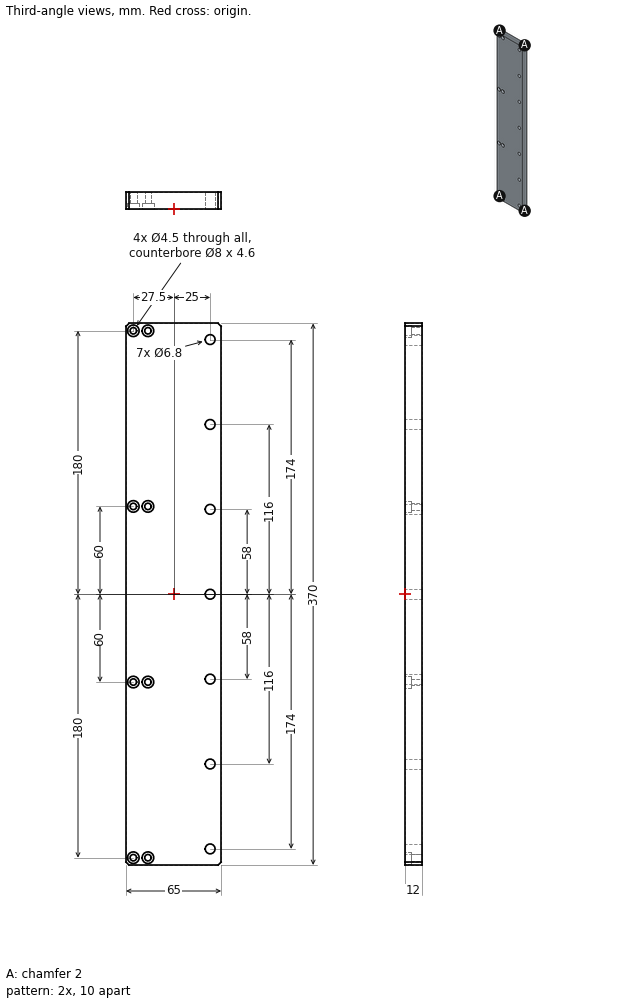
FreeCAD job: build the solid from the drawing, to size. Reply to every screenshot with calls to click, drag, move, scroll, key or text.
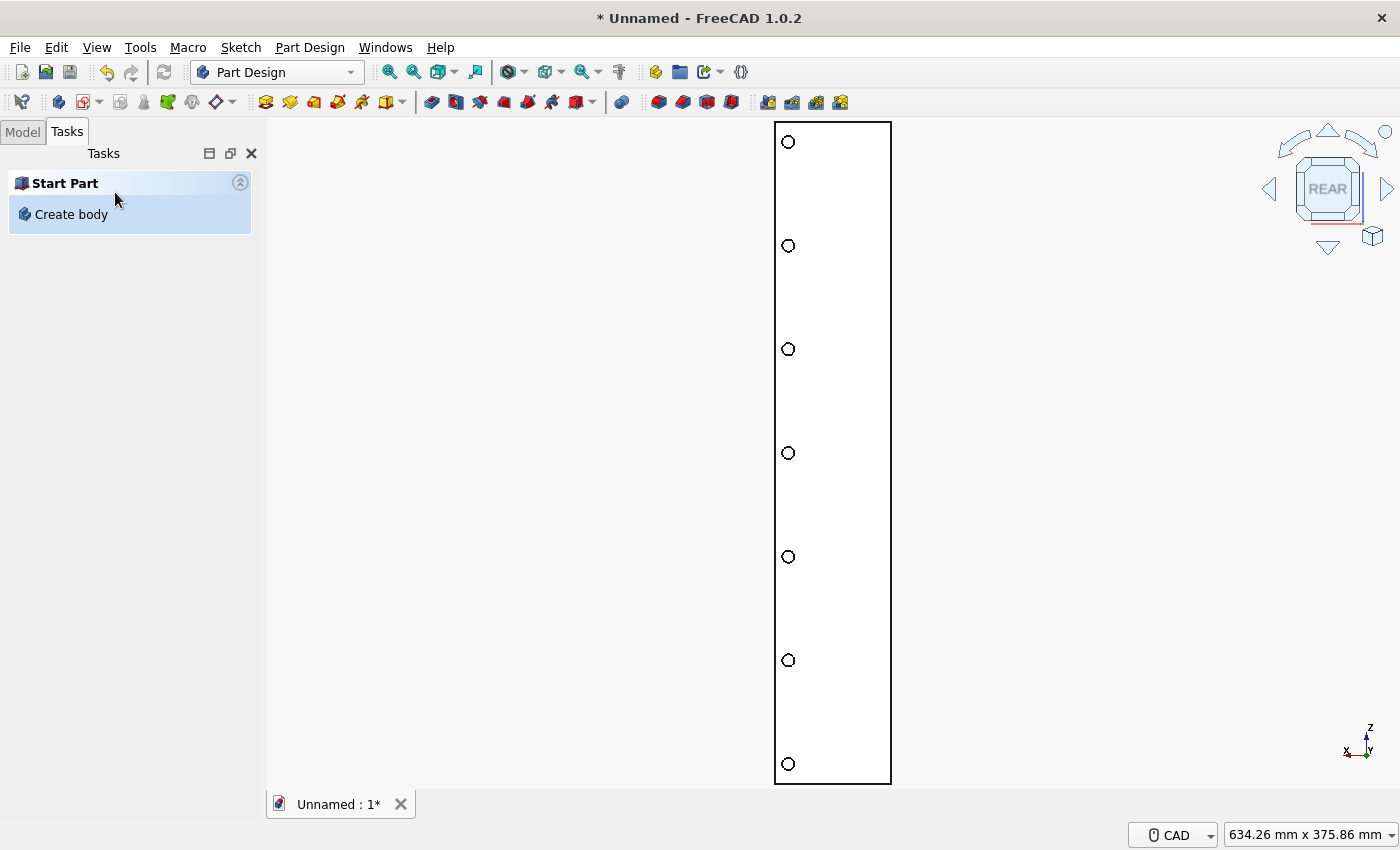
key(0)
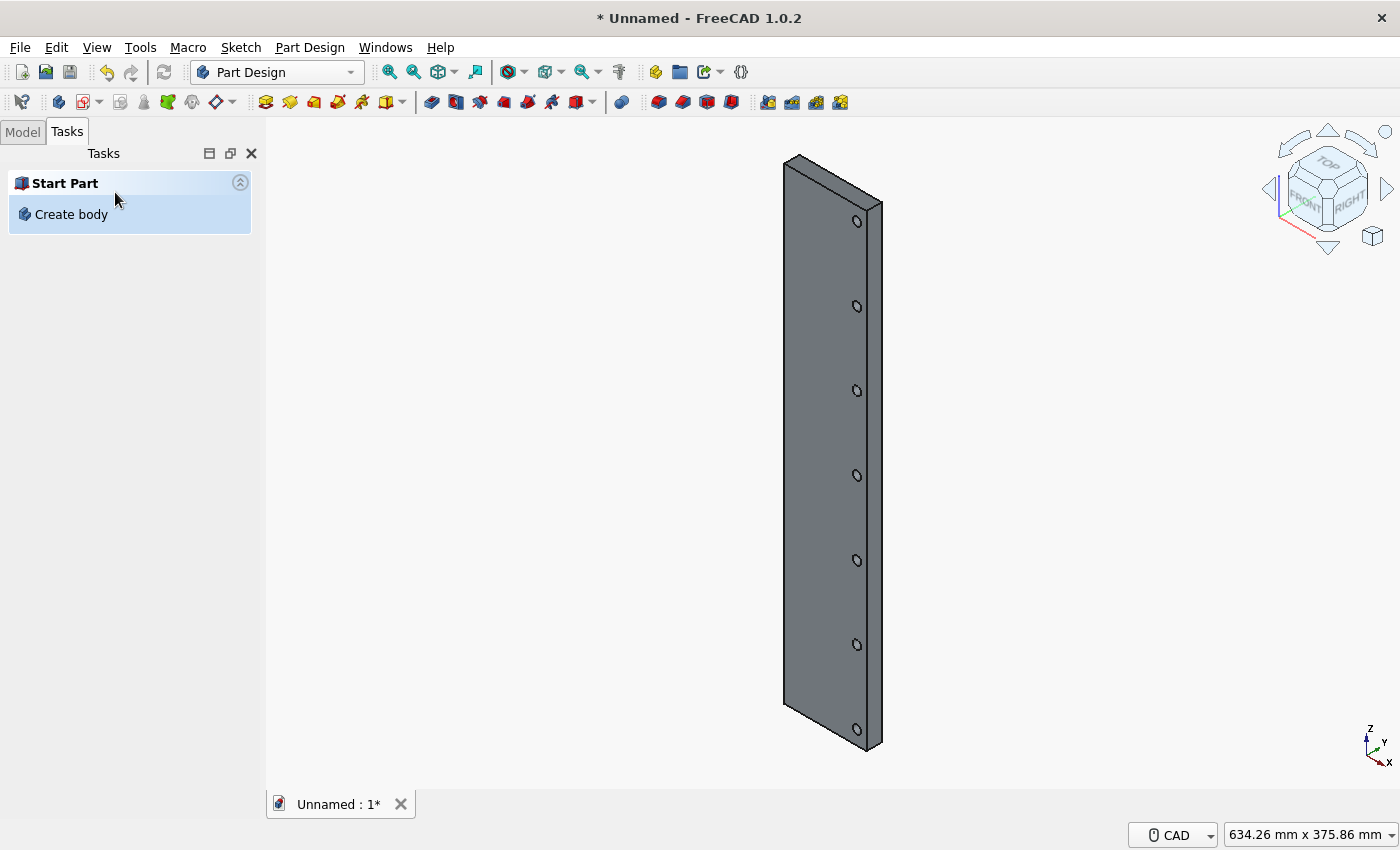
click(825, 225)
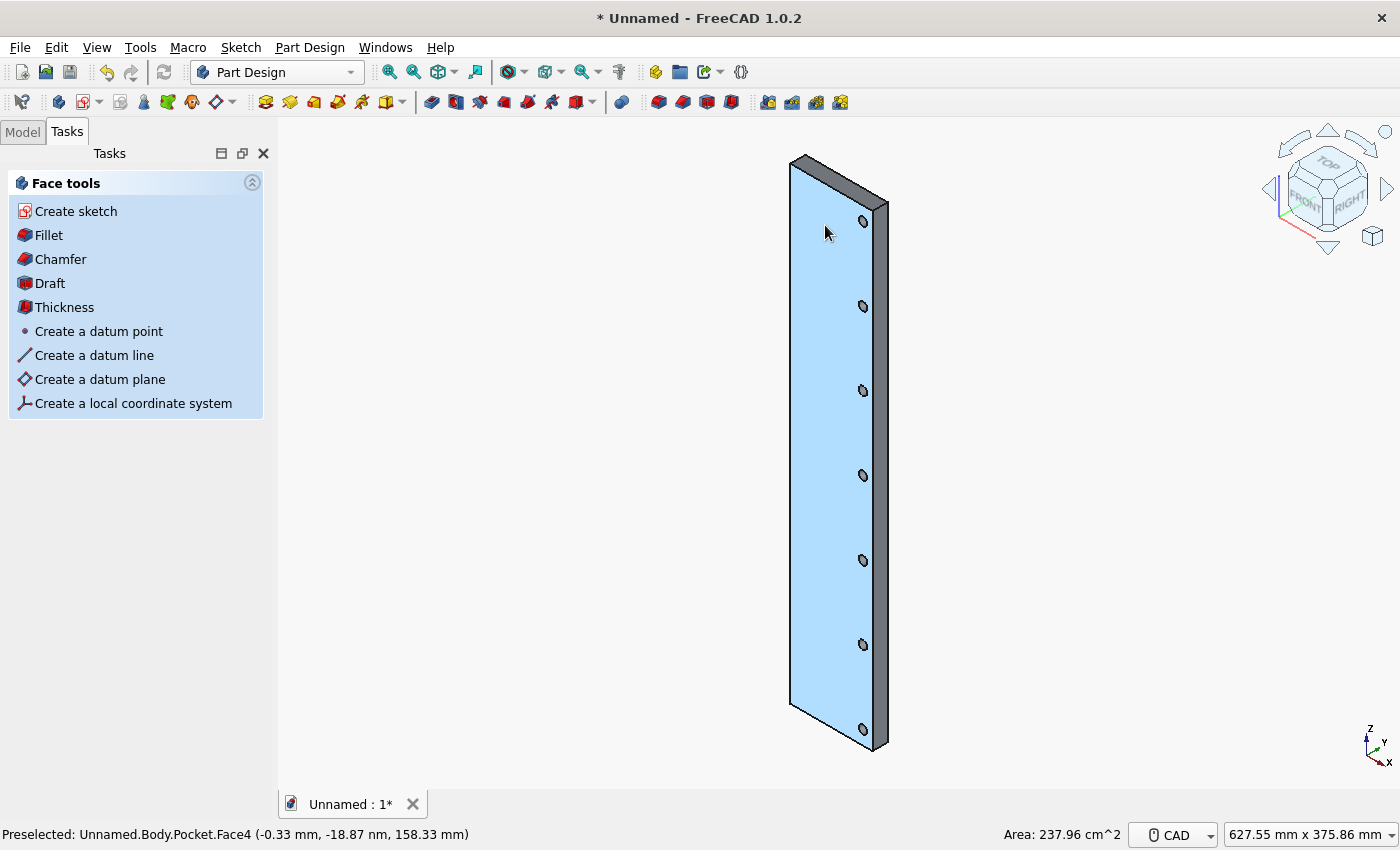
click(84, 102)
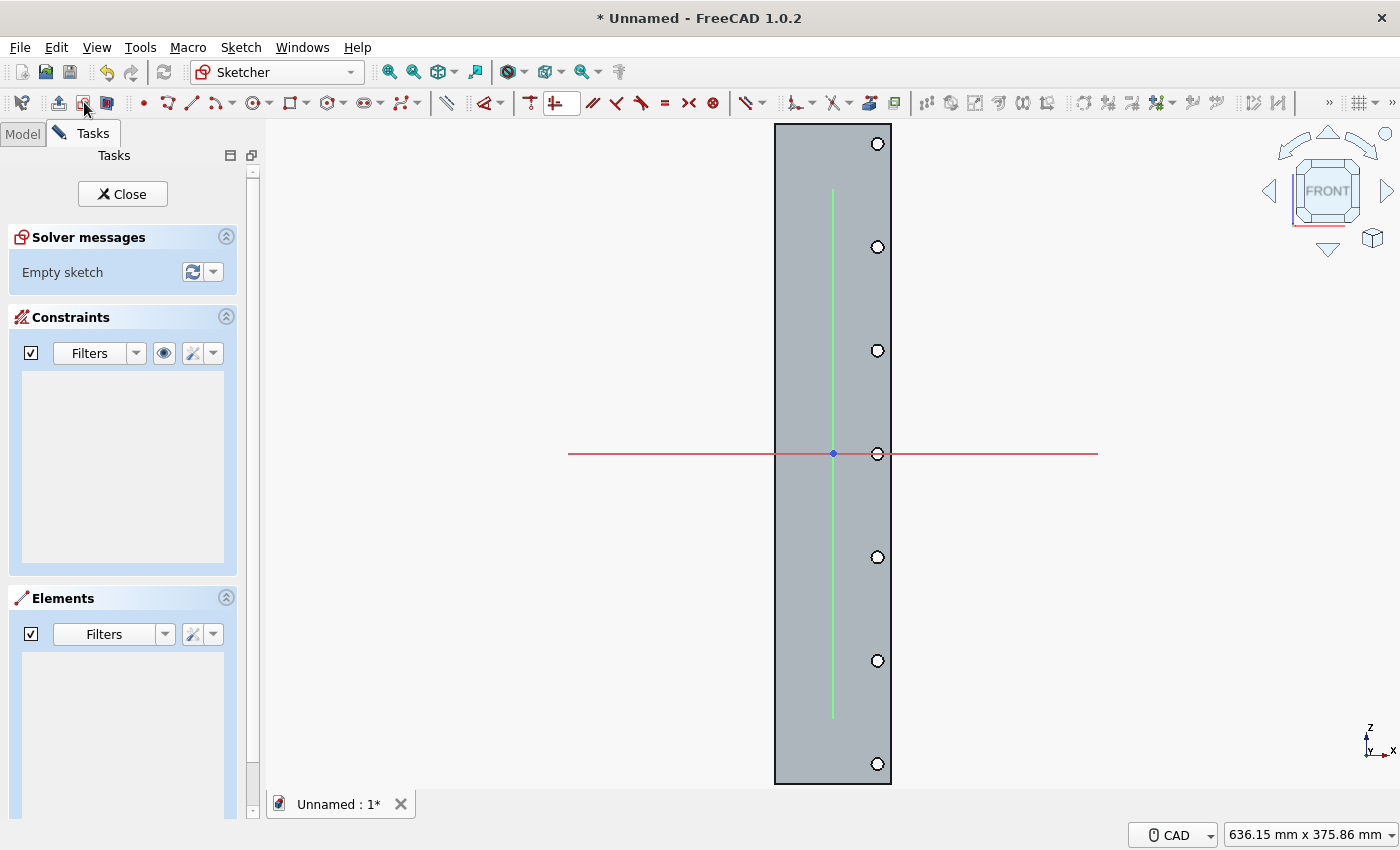
scroll(679, 454, down, 2)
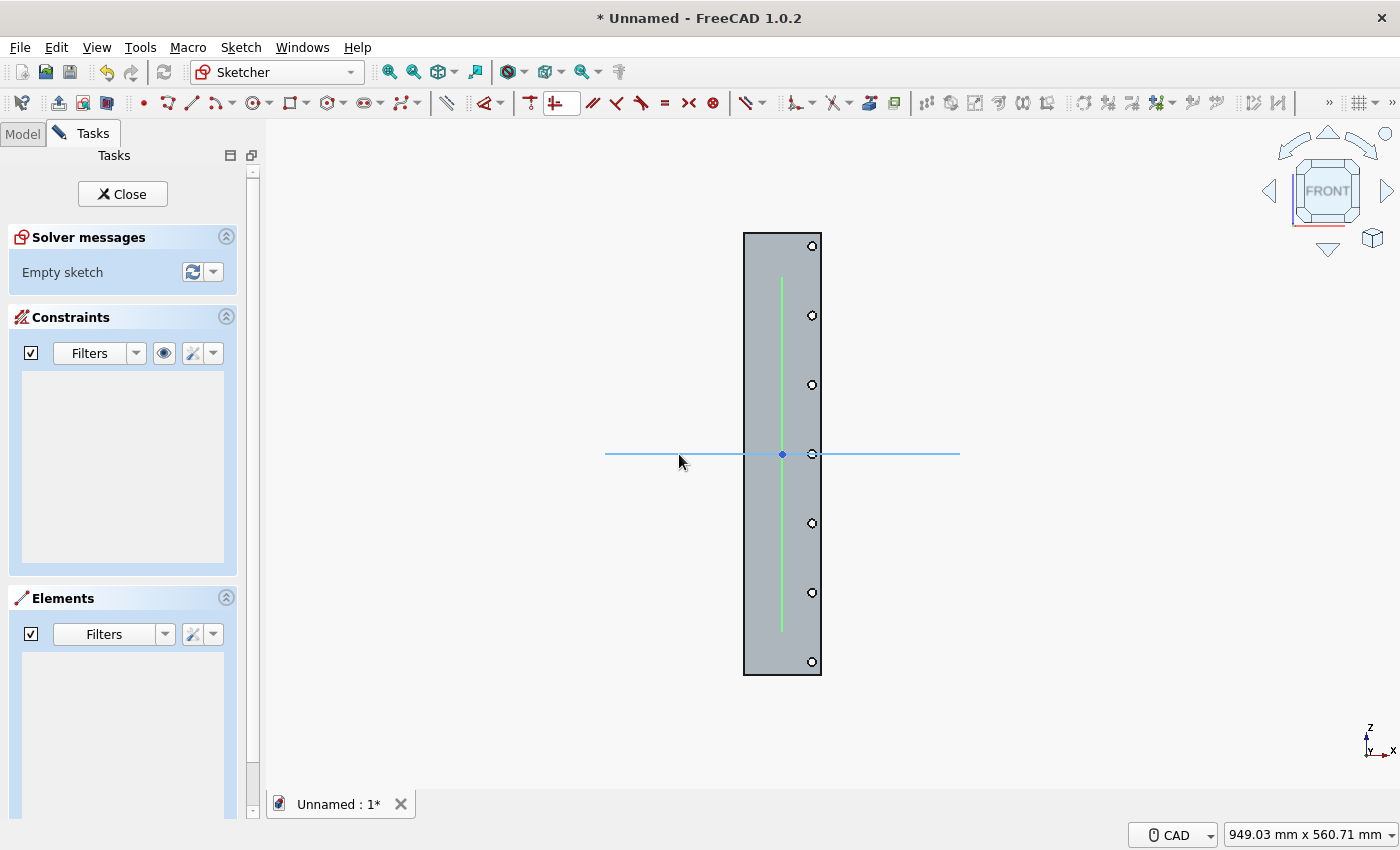
key(g)
key(c)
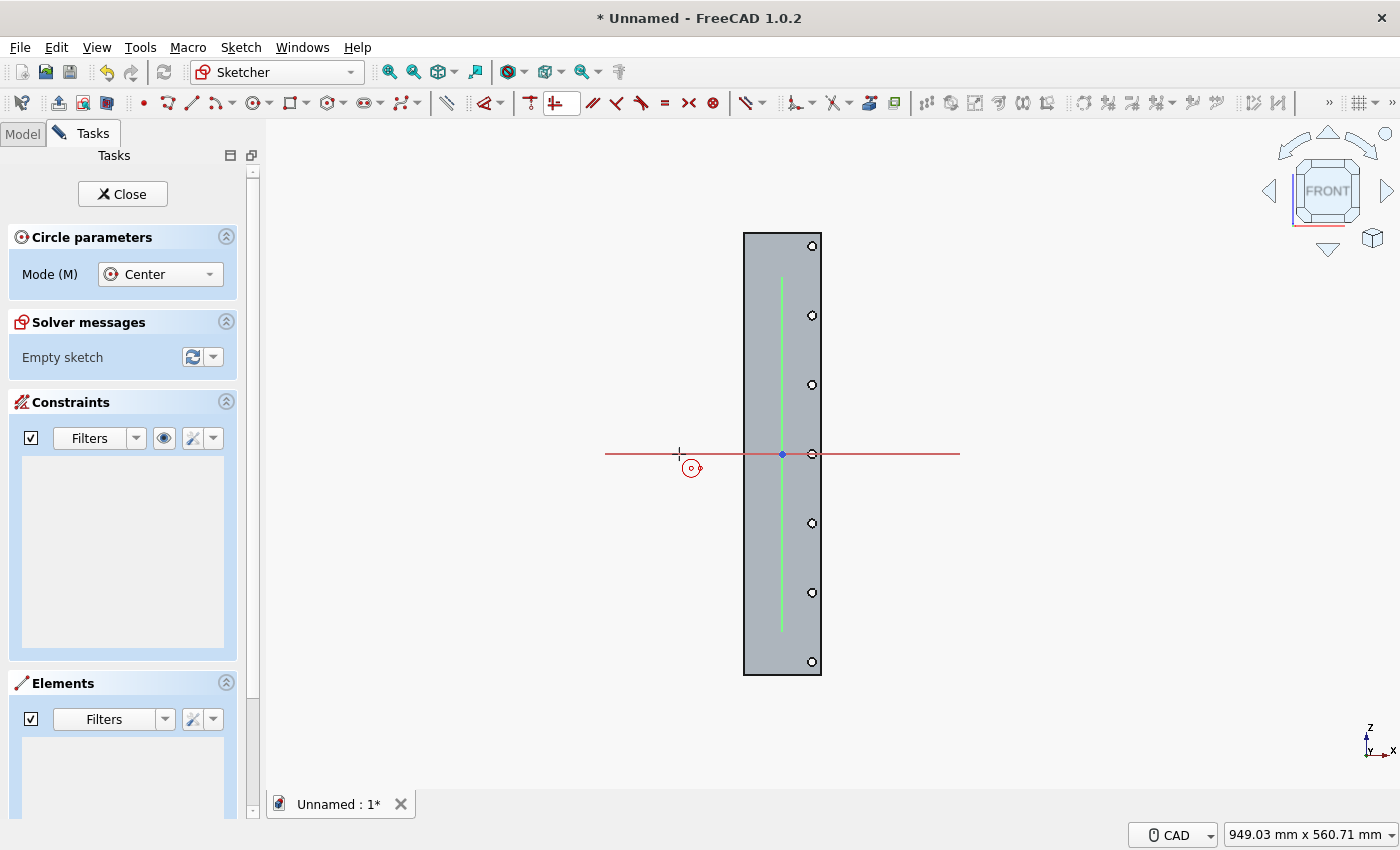
scroll(749, 239, up, 11)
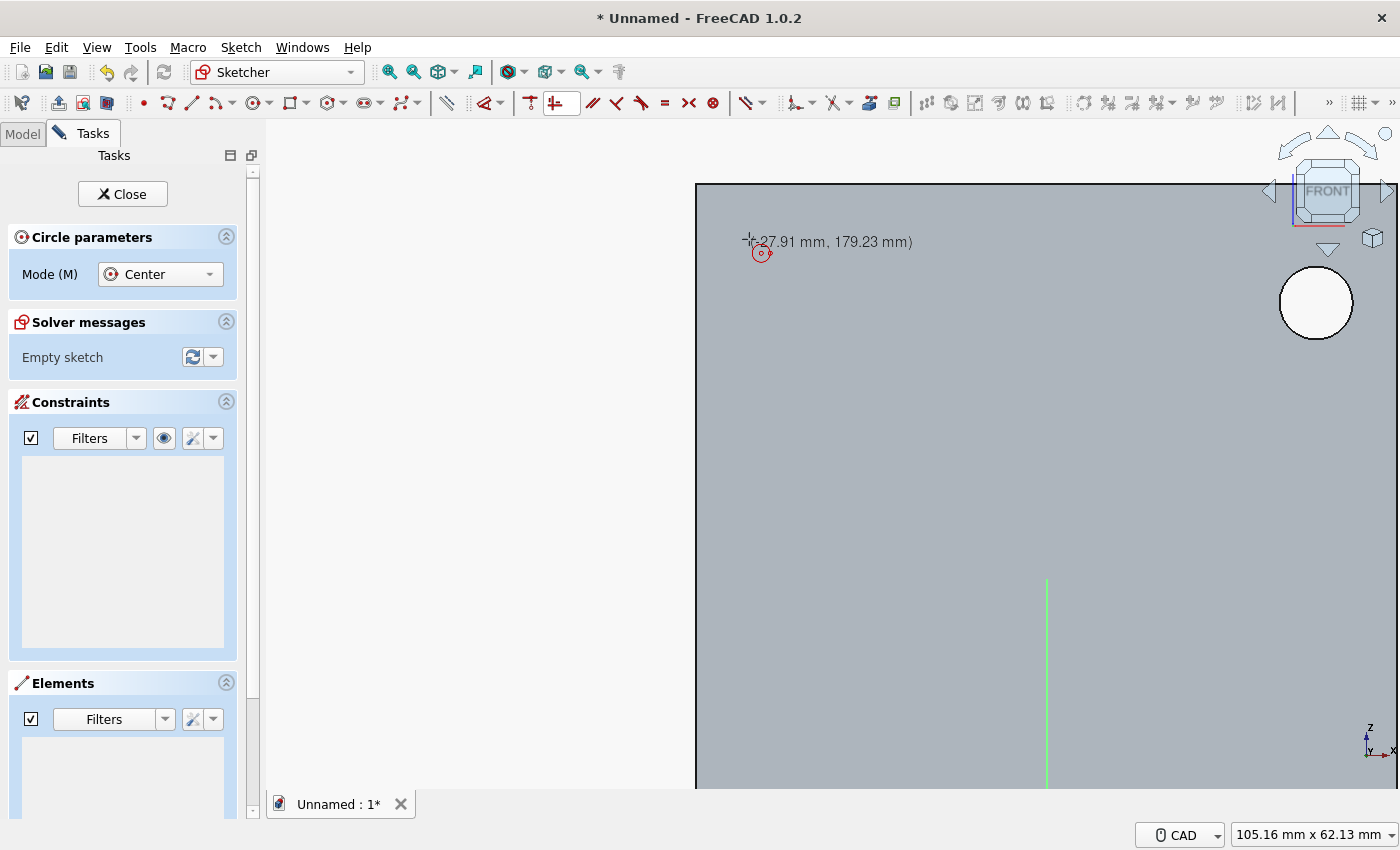
scroll(749, 239, down, 11)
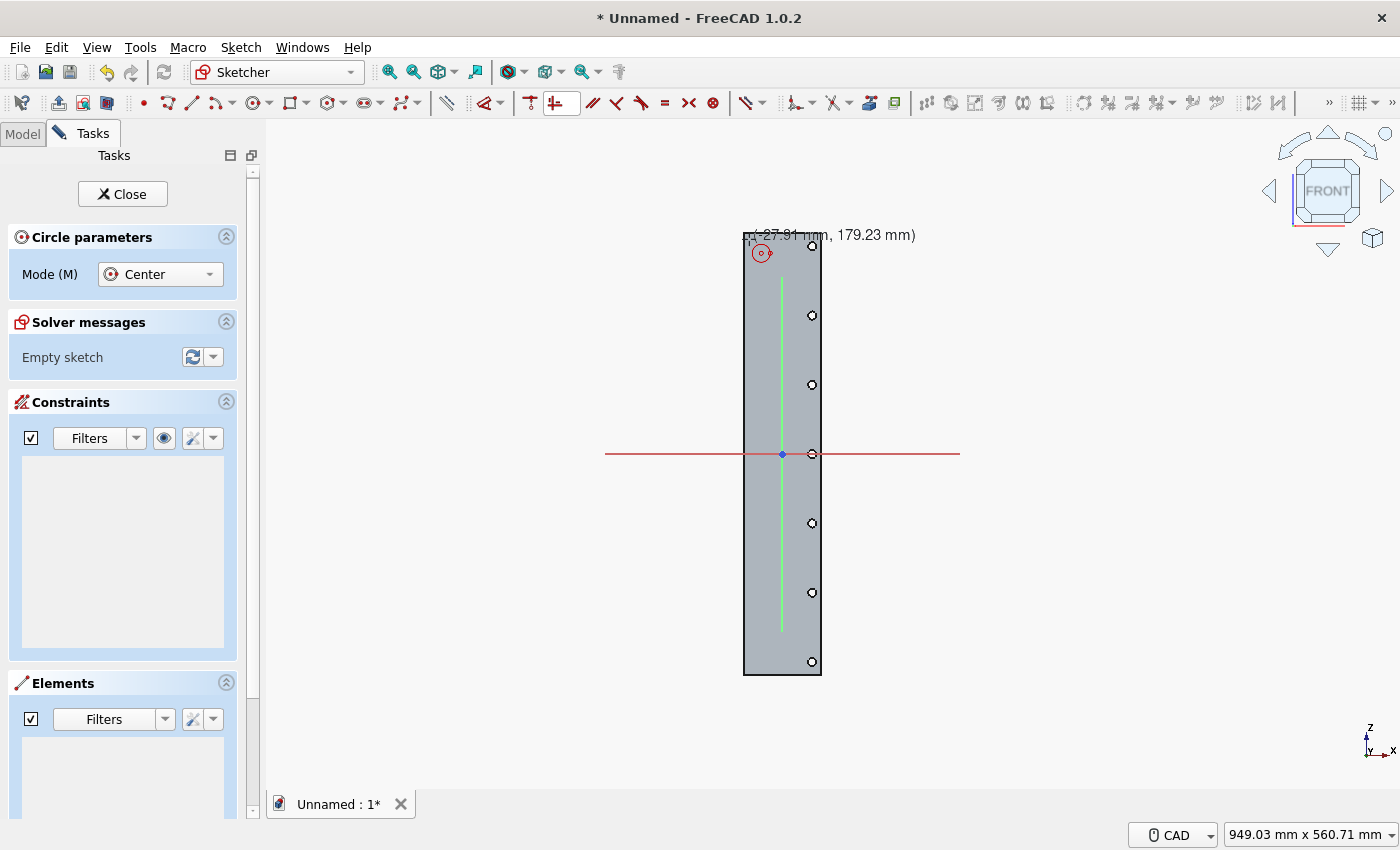
click(749, 239)
move(751, 237)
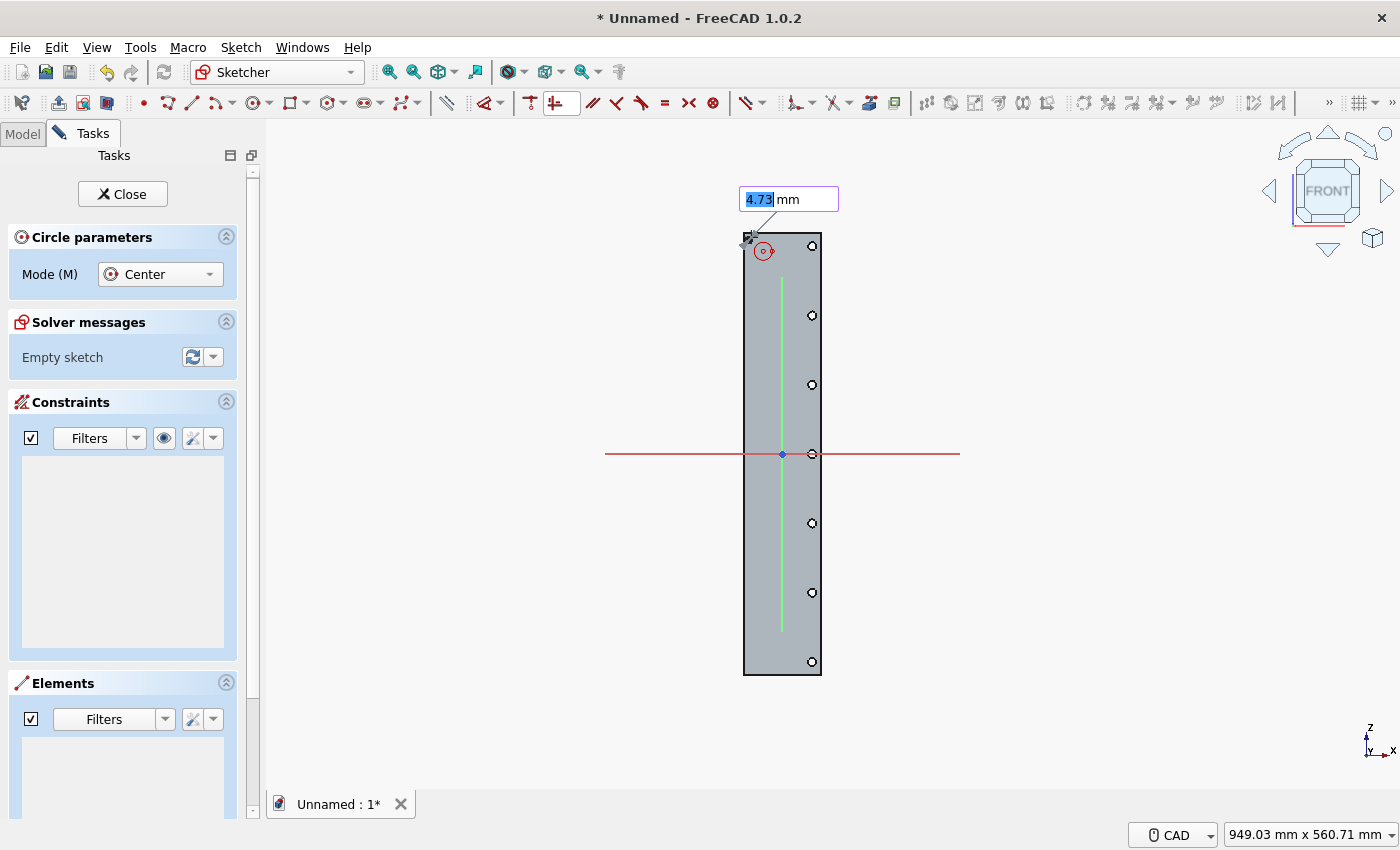
text(4.5)
key(Return)